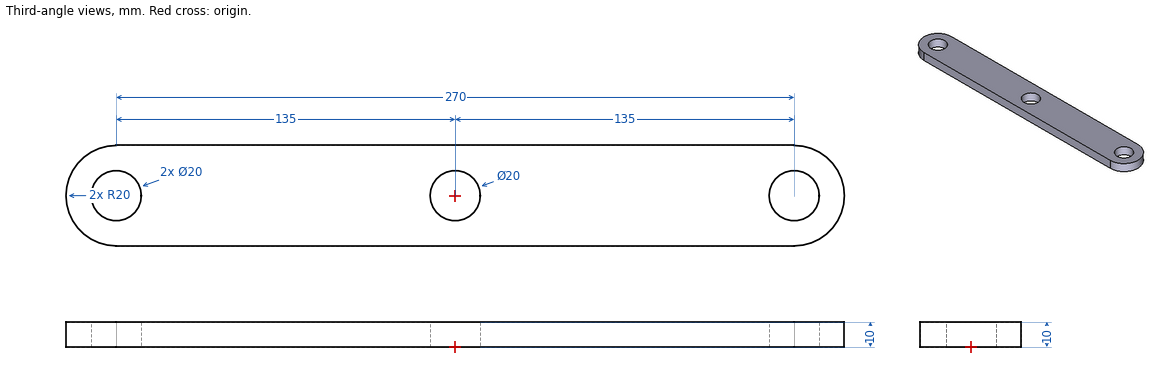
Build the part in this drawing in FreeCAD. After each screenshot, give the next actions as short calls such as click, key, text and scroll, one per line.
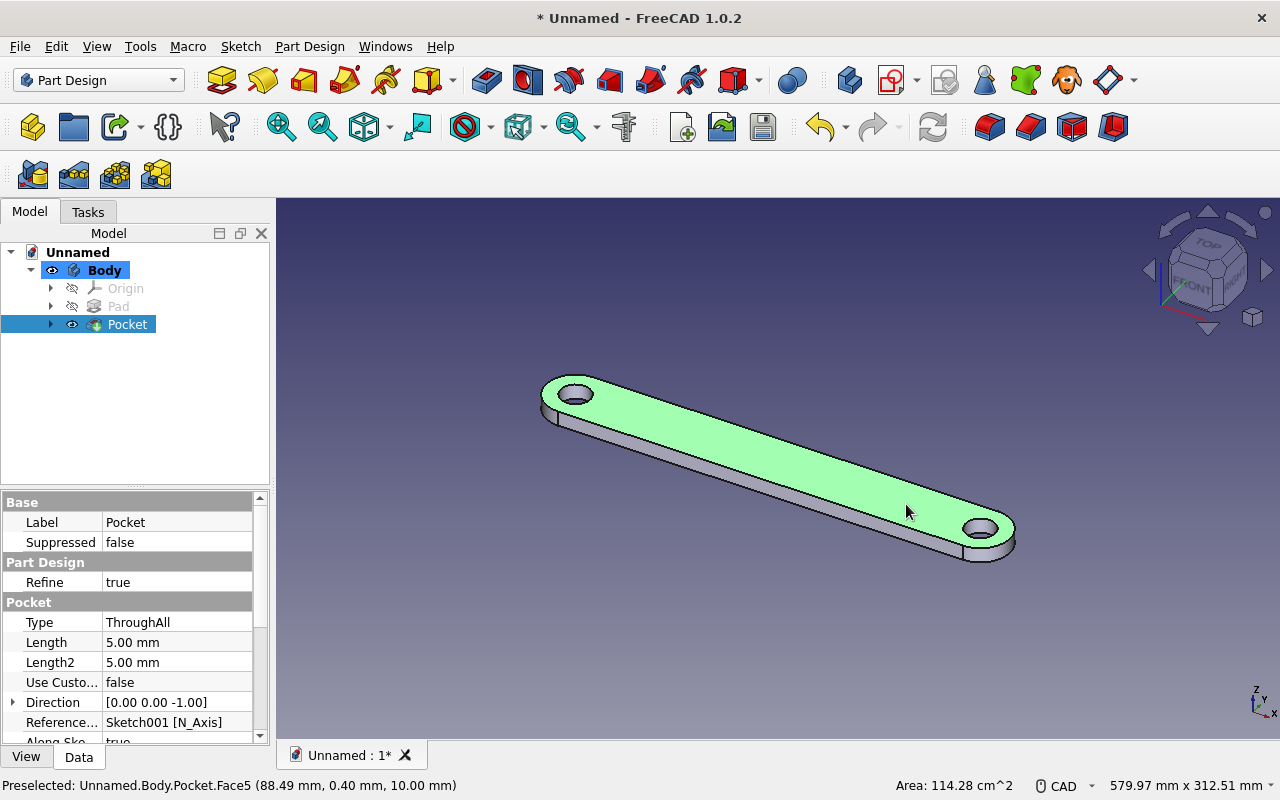
click(890, 80)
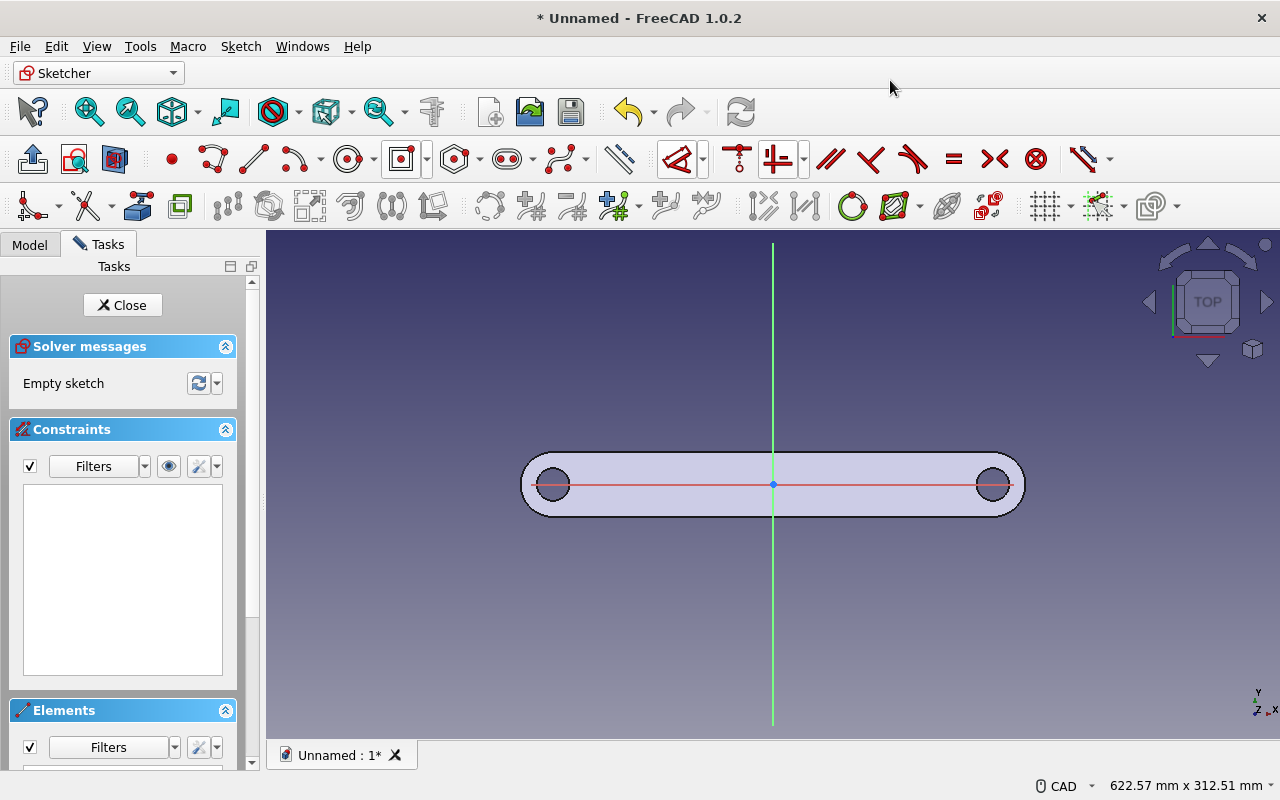
scroll(782, 485, up, 11)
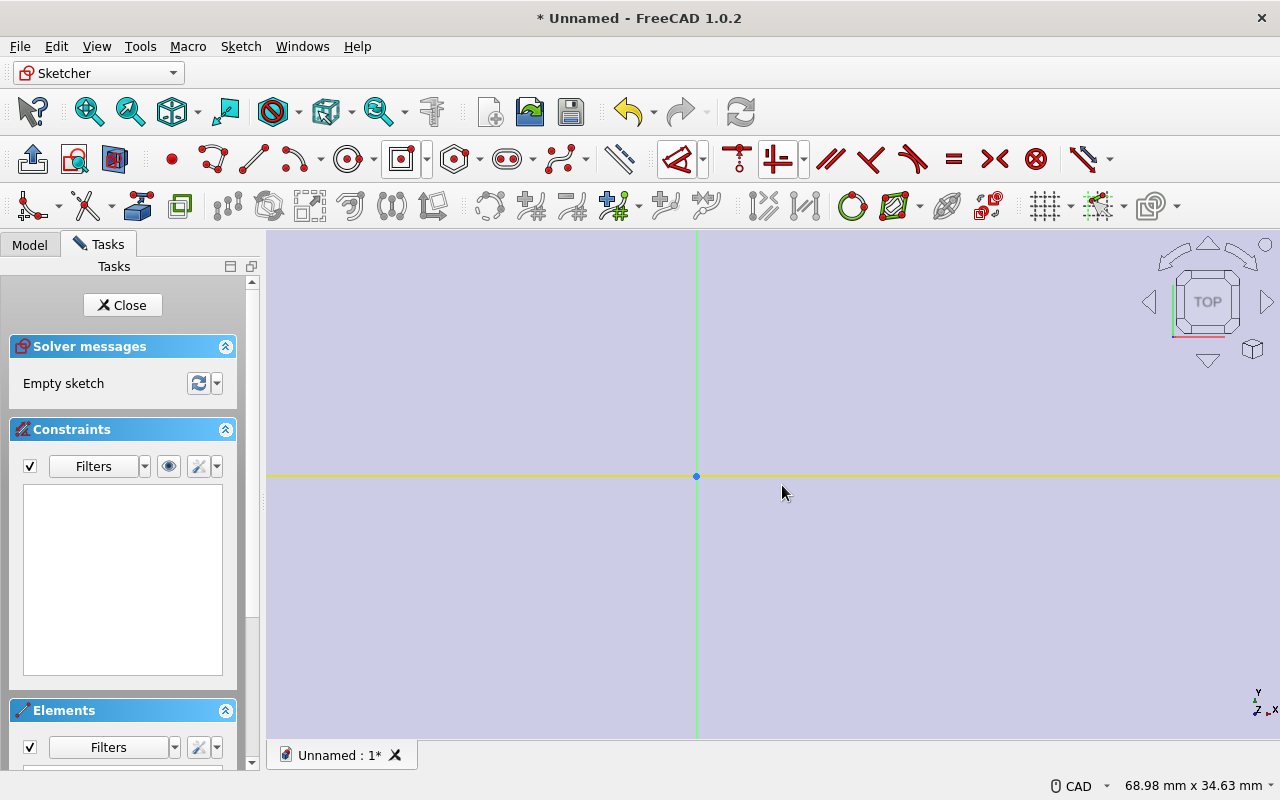
click(348, 160)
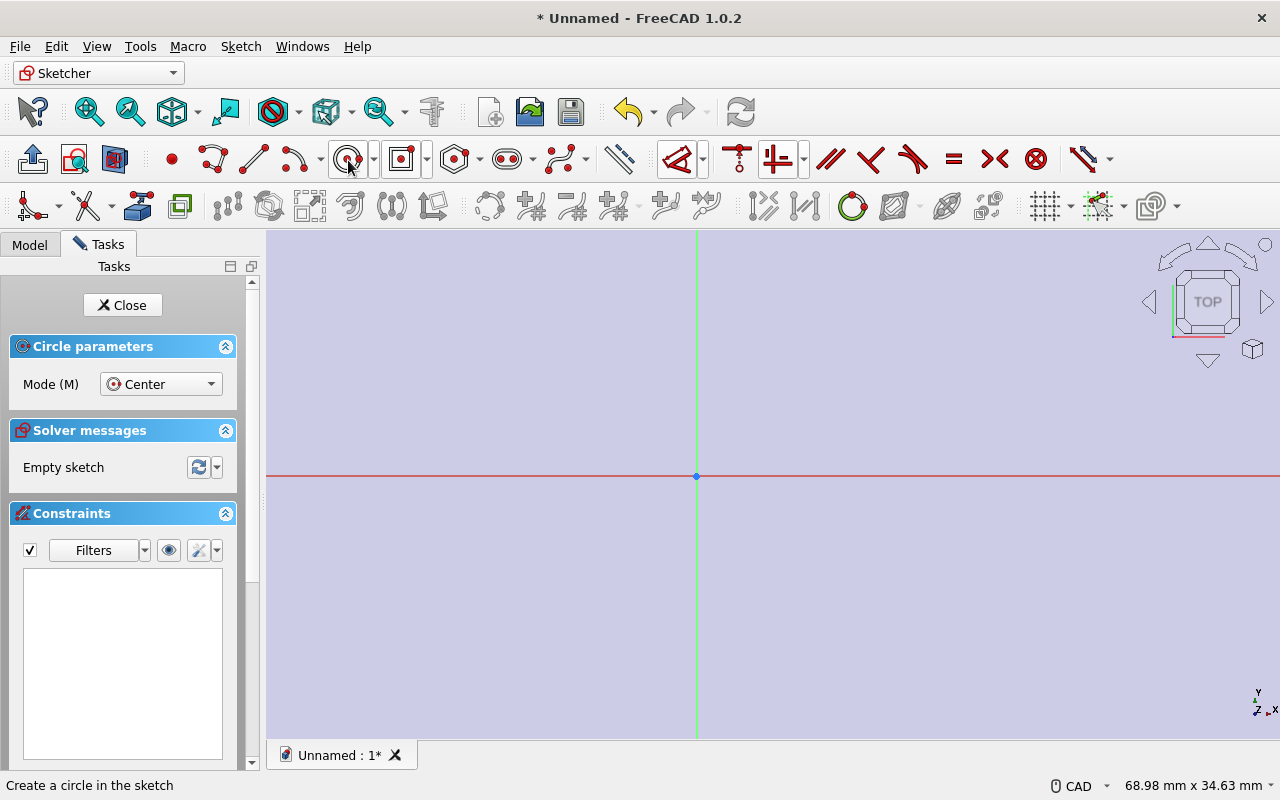
click(697, 476)
click(801, 373)
key(Escape)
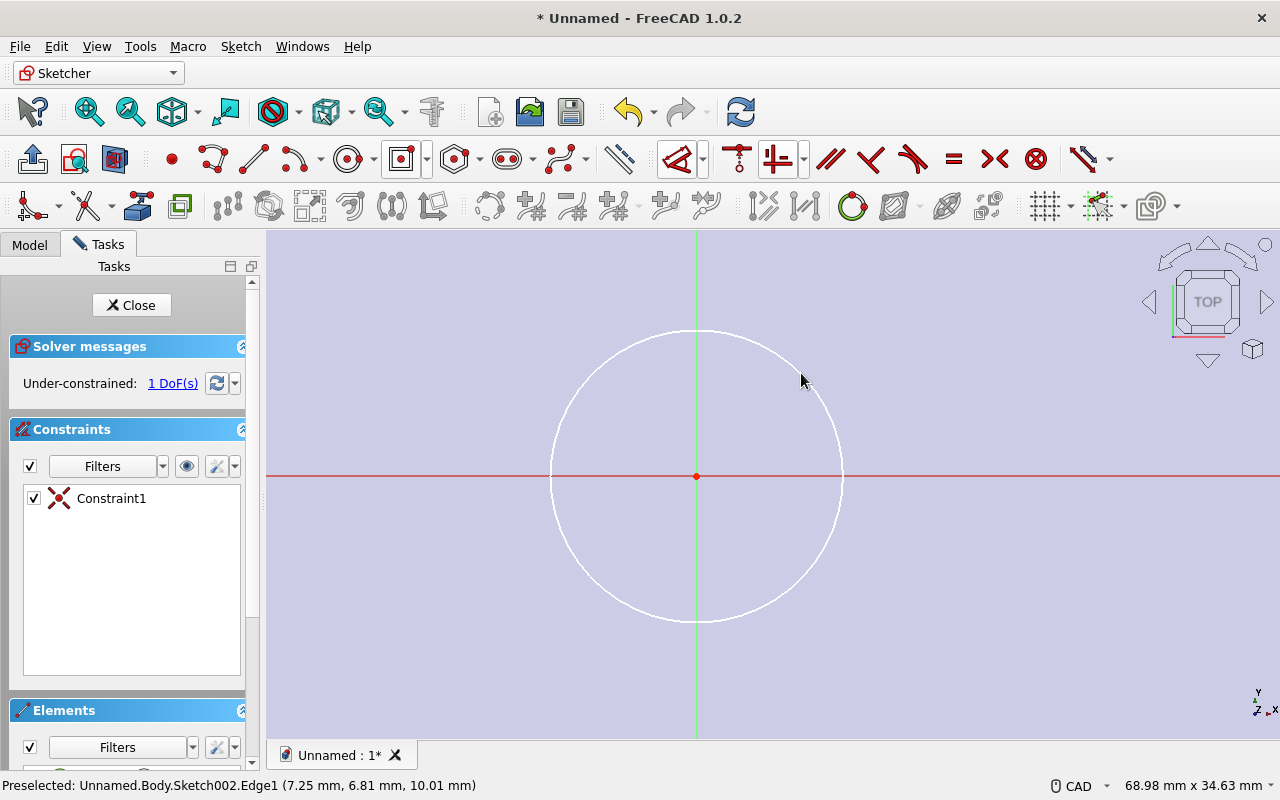
click(800, 373)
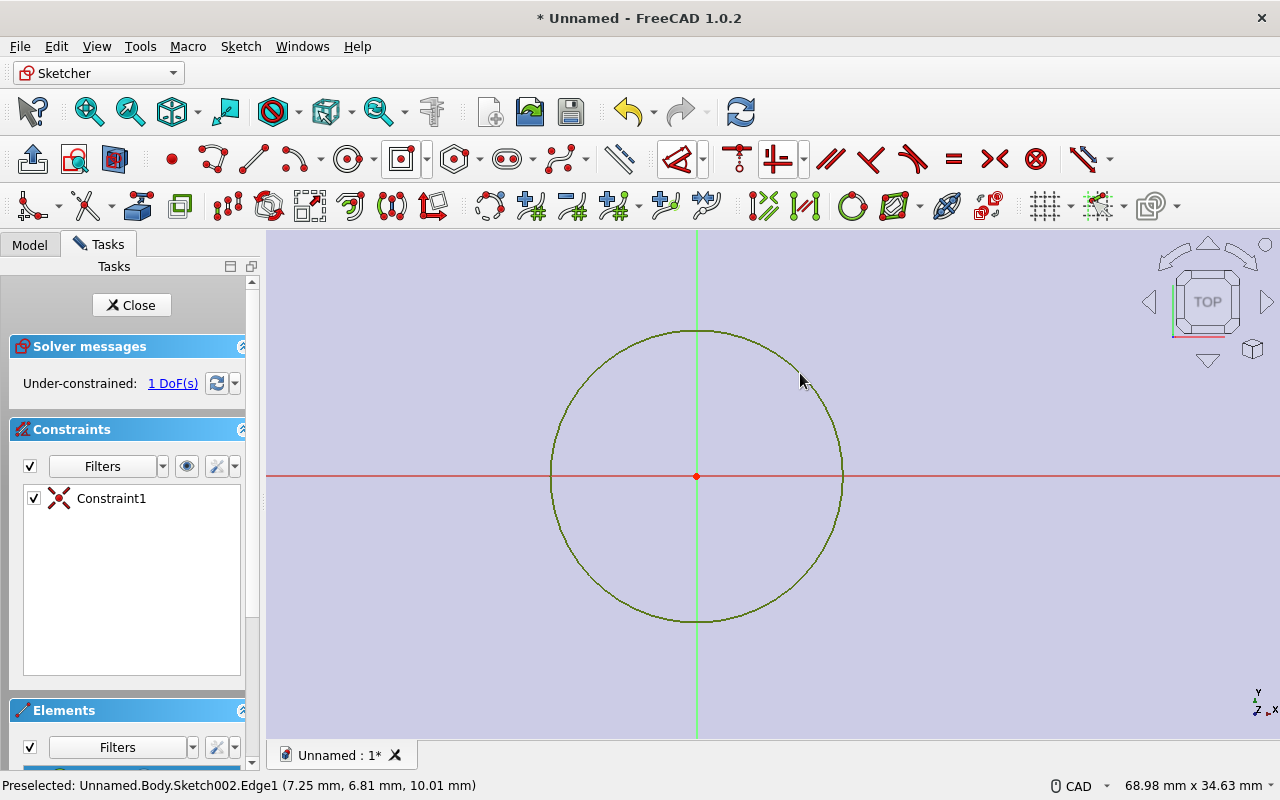
click(702, 160)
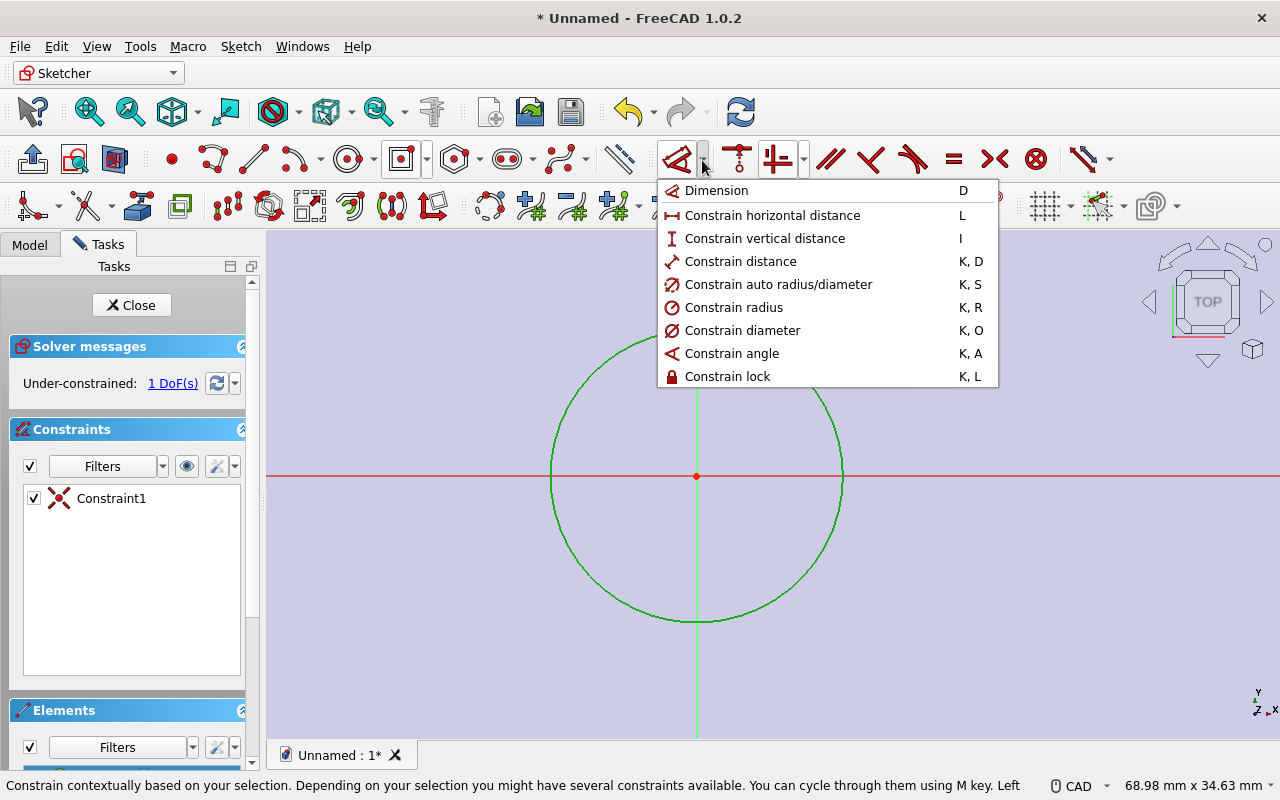
click(828, 330)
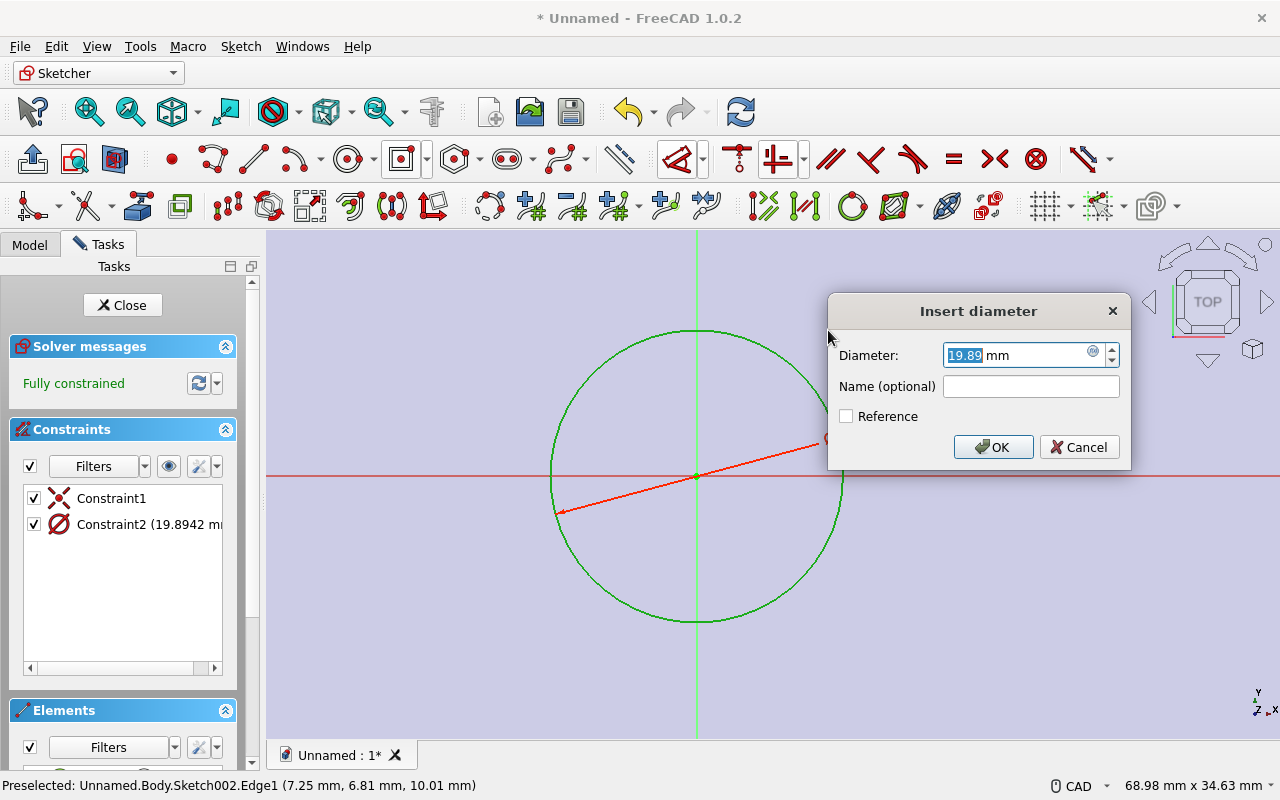
text(20)
key(Return)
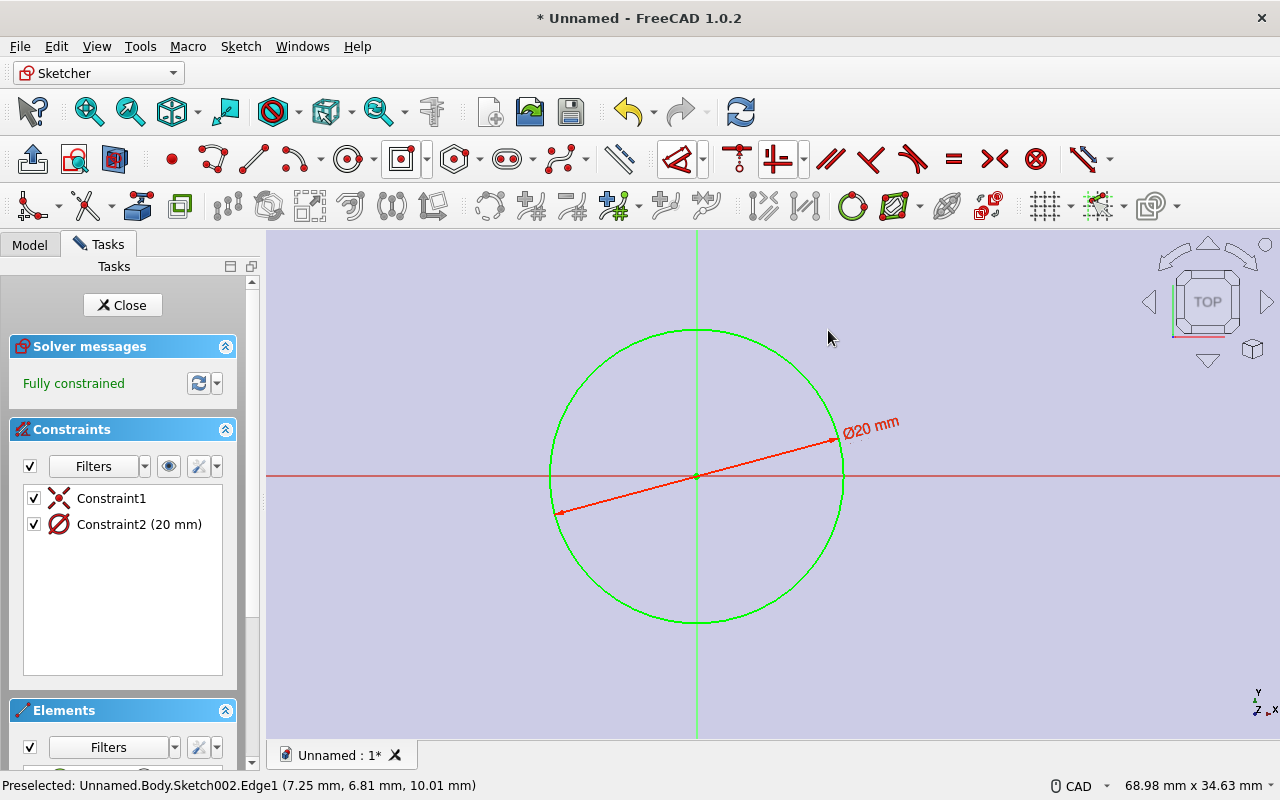
click(123, 305)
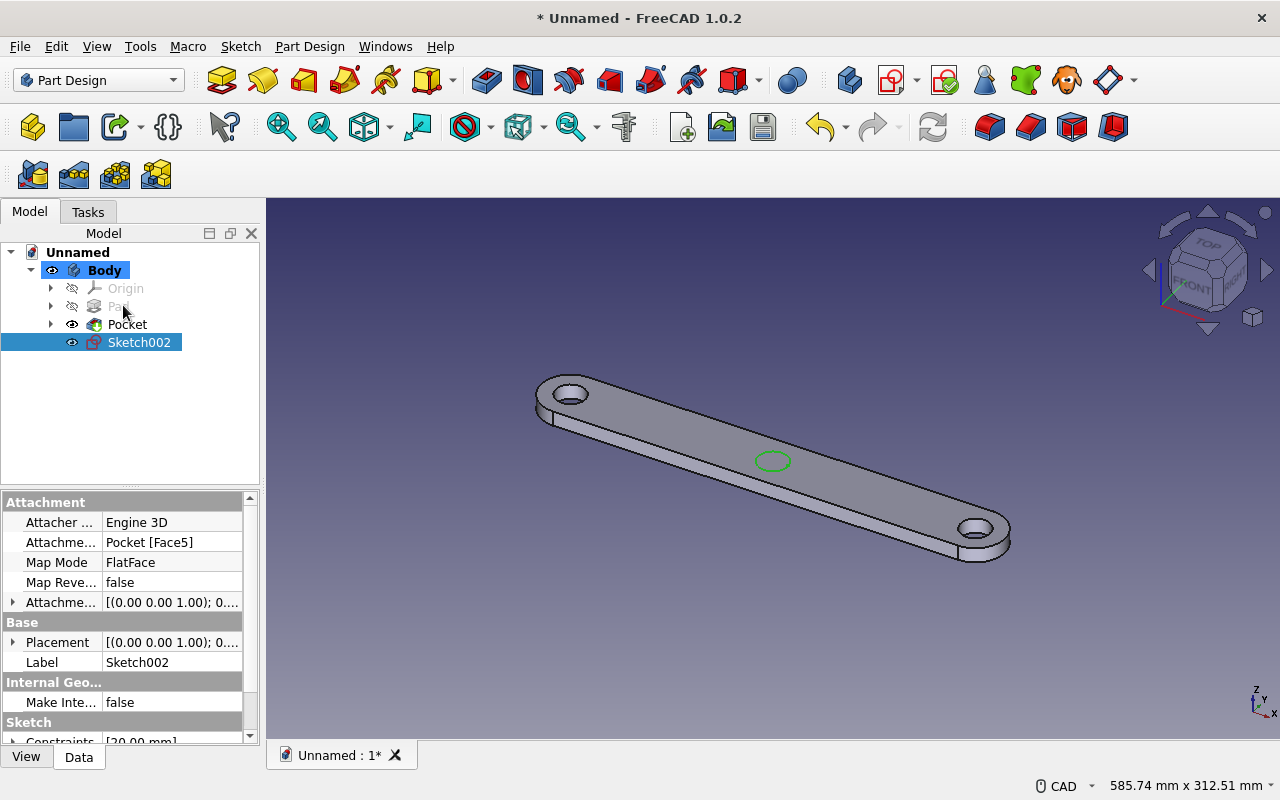
click(487, 80)